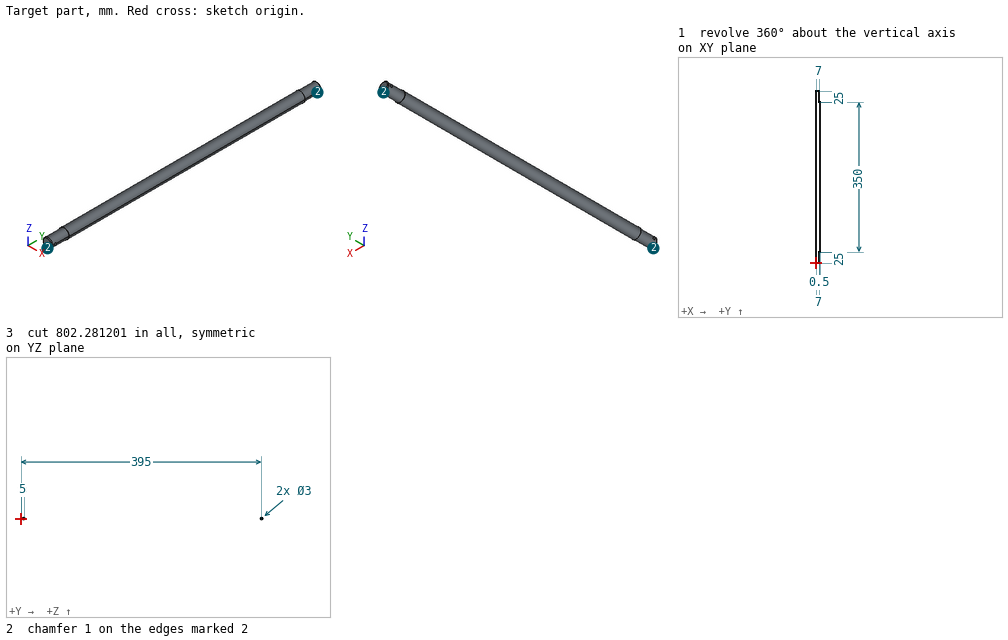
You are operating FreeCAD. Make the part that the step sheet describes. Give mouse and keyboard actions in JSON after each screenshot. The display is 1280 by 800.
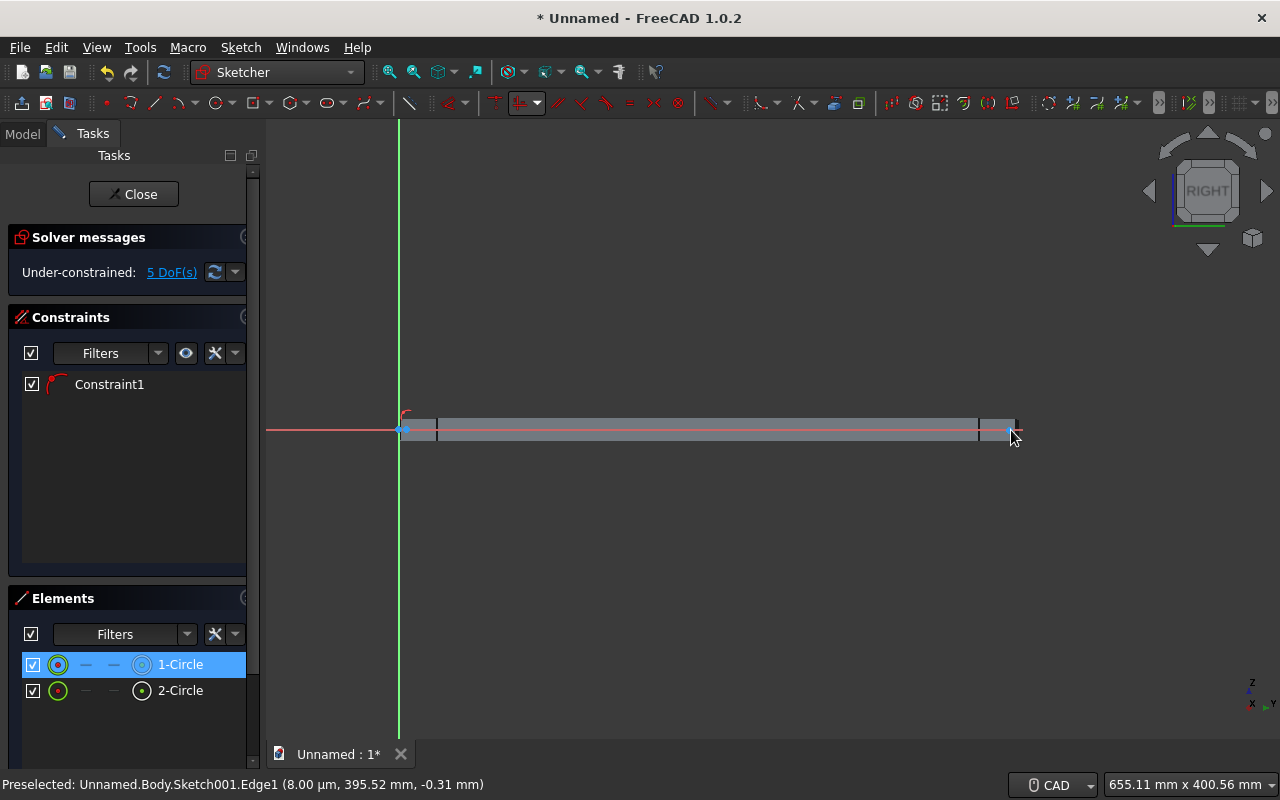
{"action": "scroll", "coordinate": [408, 428], "scroll_direction": "up", "scroll_amount": 12}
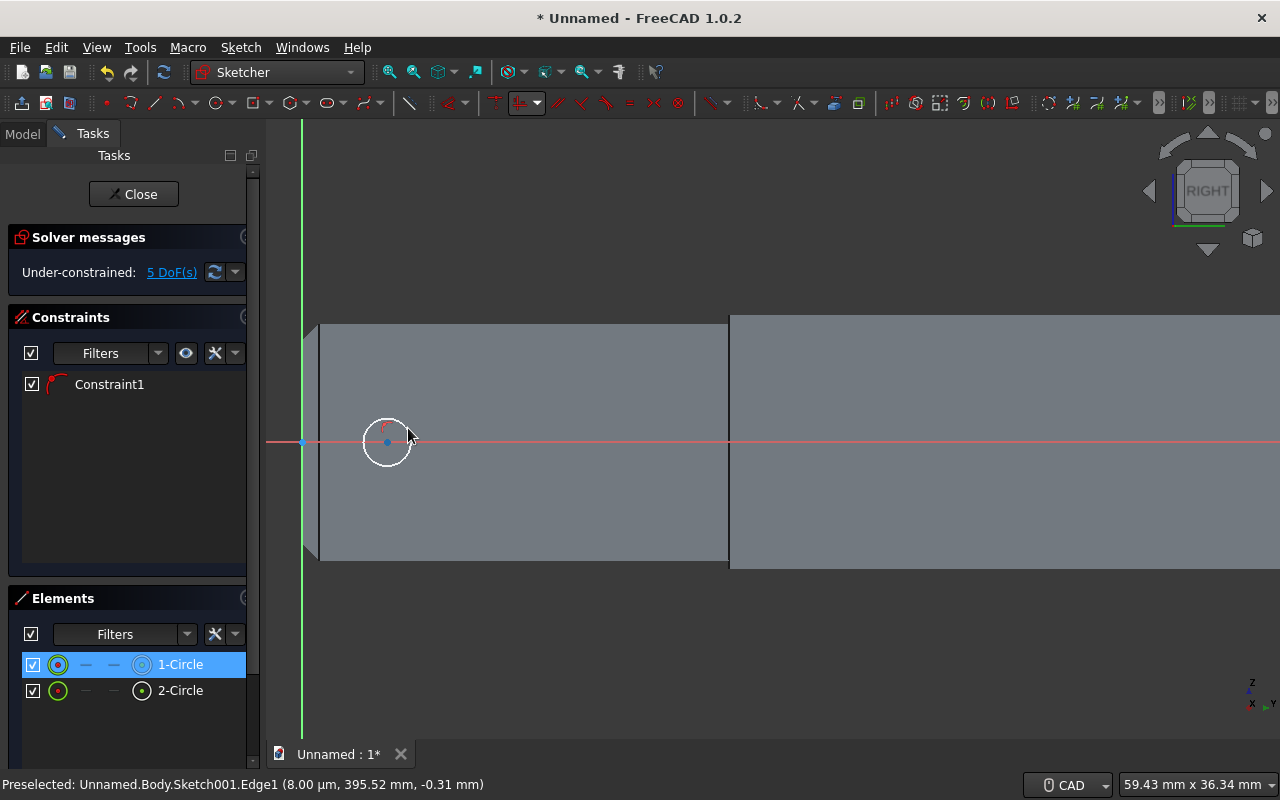
{"action": "left_click", "coordinate": [404, 425]}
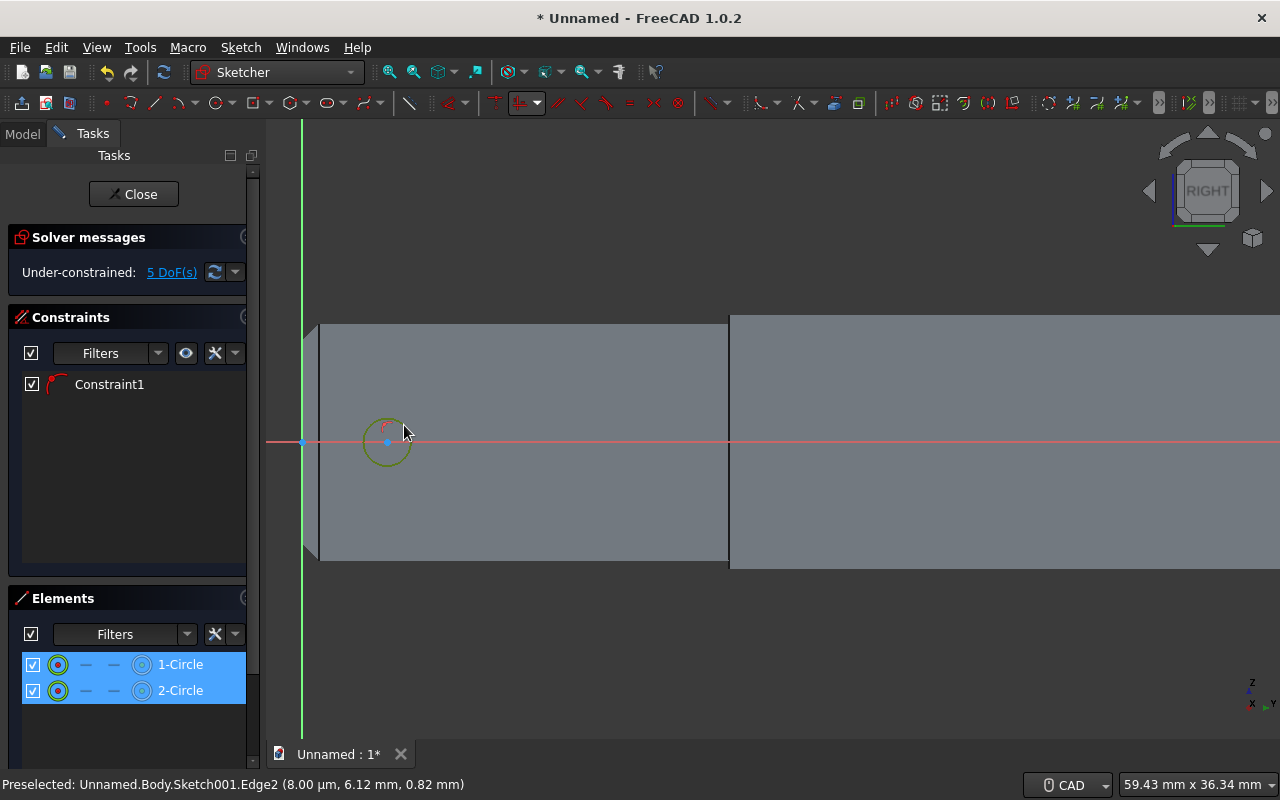
{"action": "left_click", "coordinate": [630, 104]}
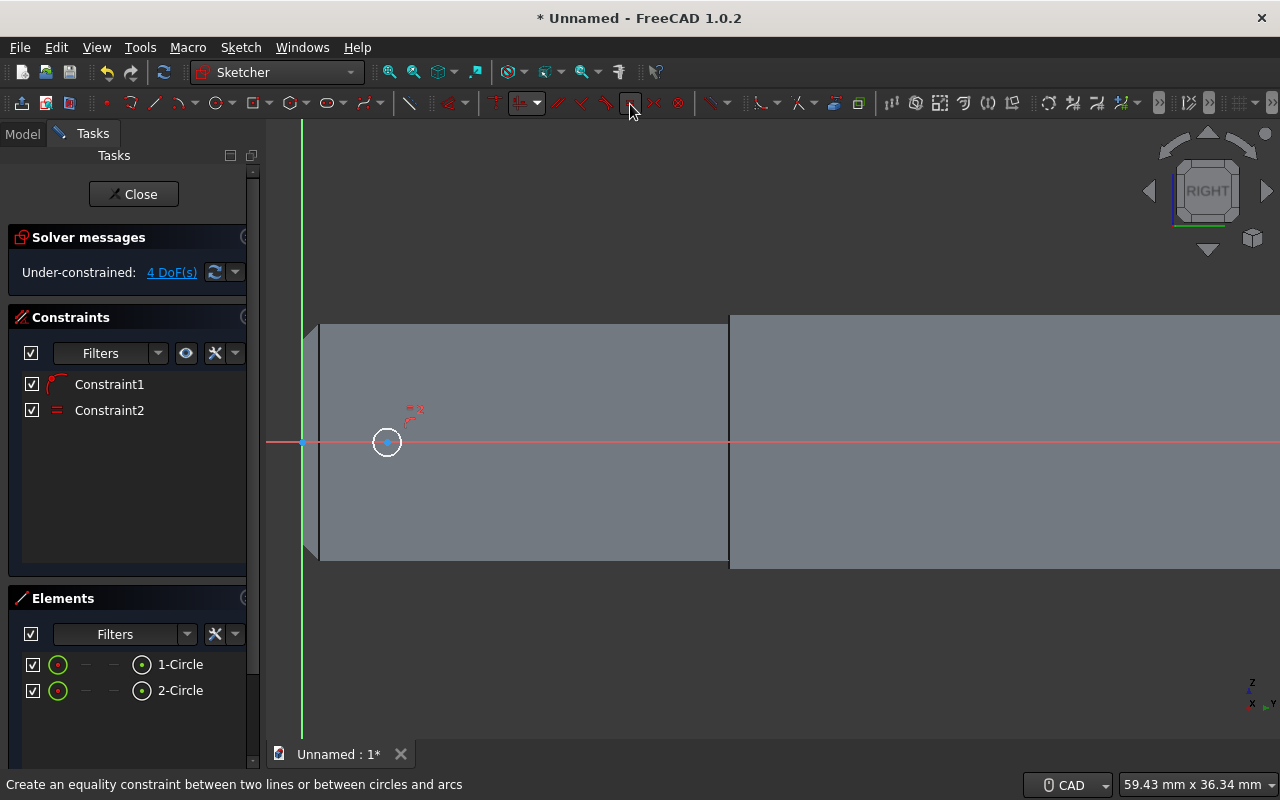
{"action": "scroll", "coordinate": [407, 428], "scroll_direction": "down", "scroll_amount": 12}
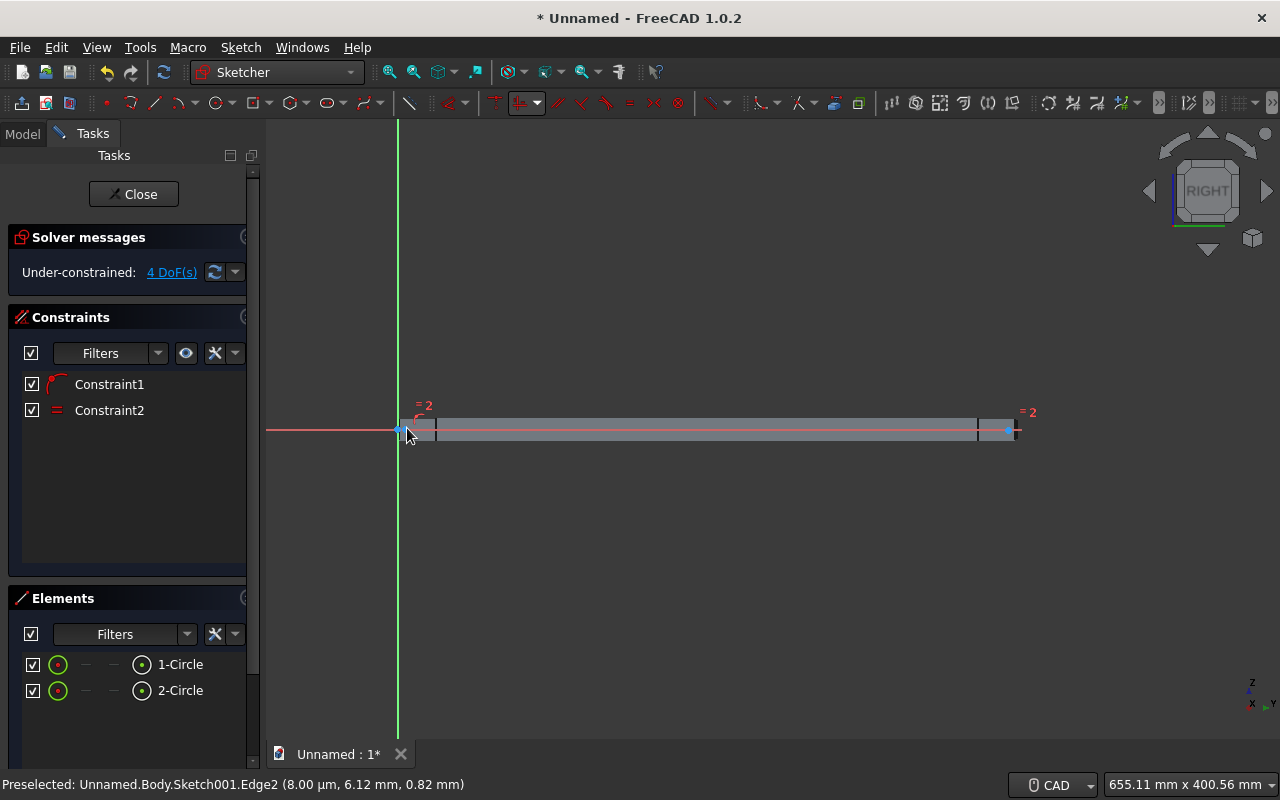
{"action": "left_click", "coordinate": [1009, 431]}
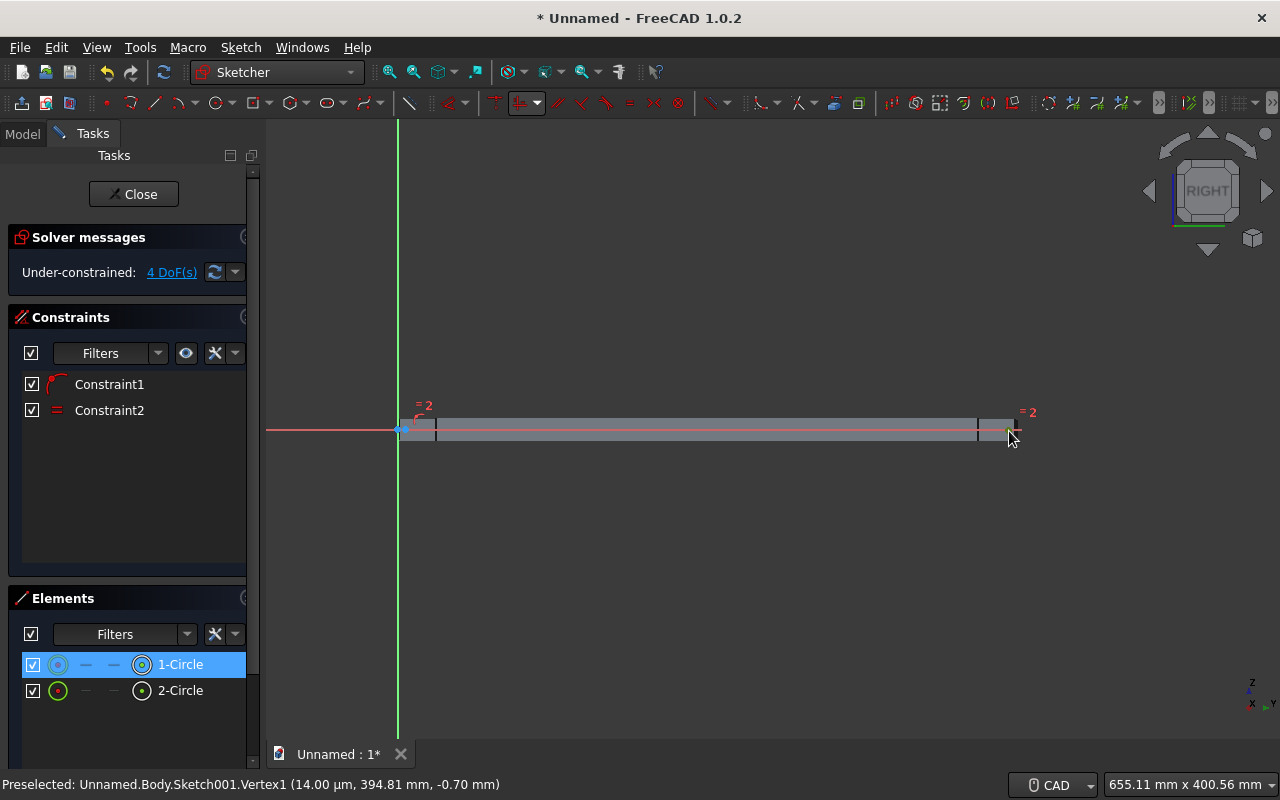
{"action": "left_click", "coordinate": [353, 430]}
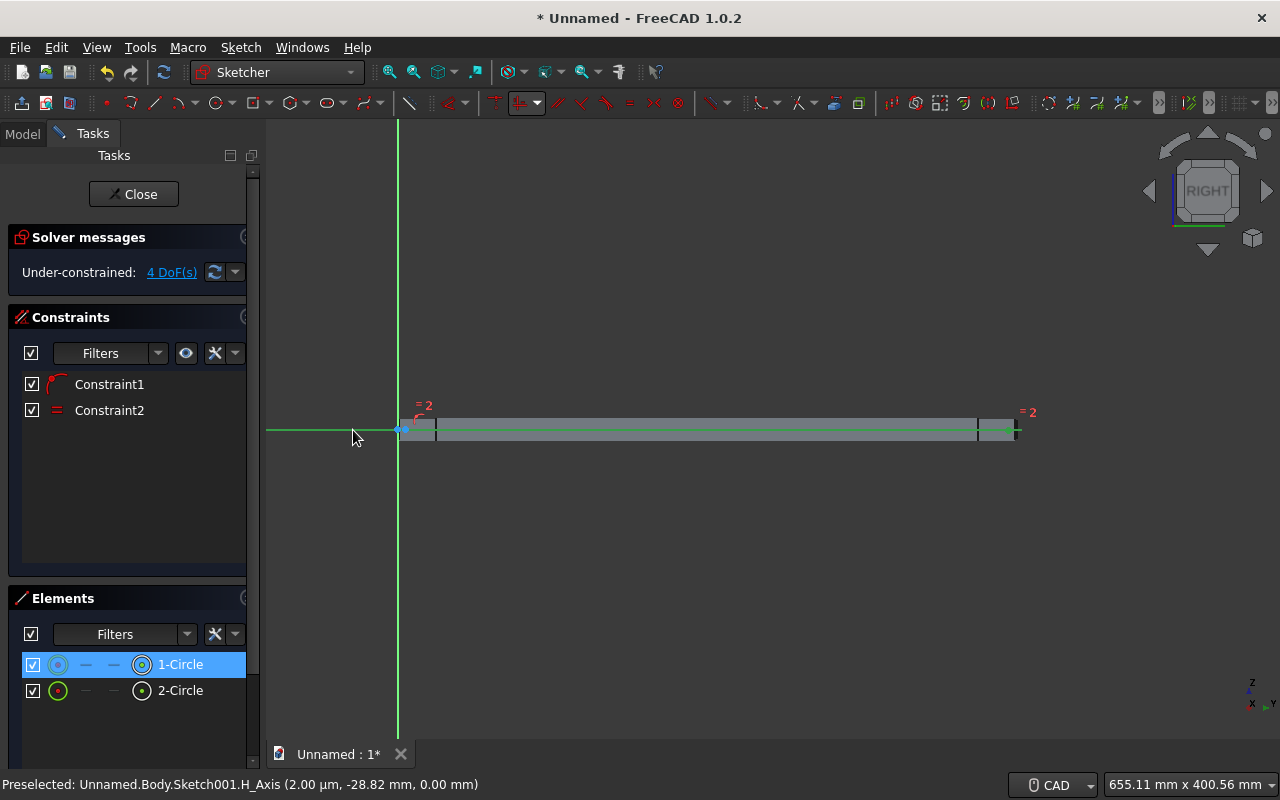
{"action": "key", "text": "c"}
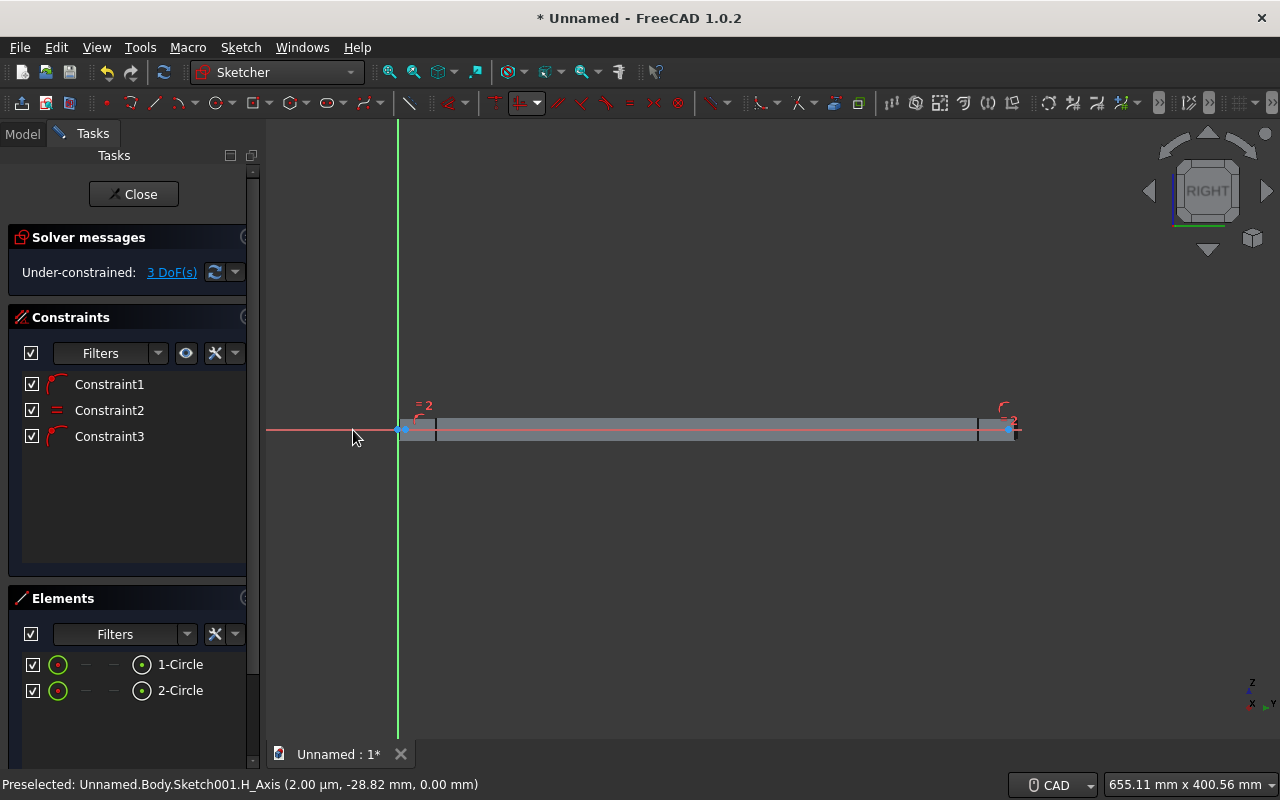
{"action": "left_click", "coordinate": [448, 104]}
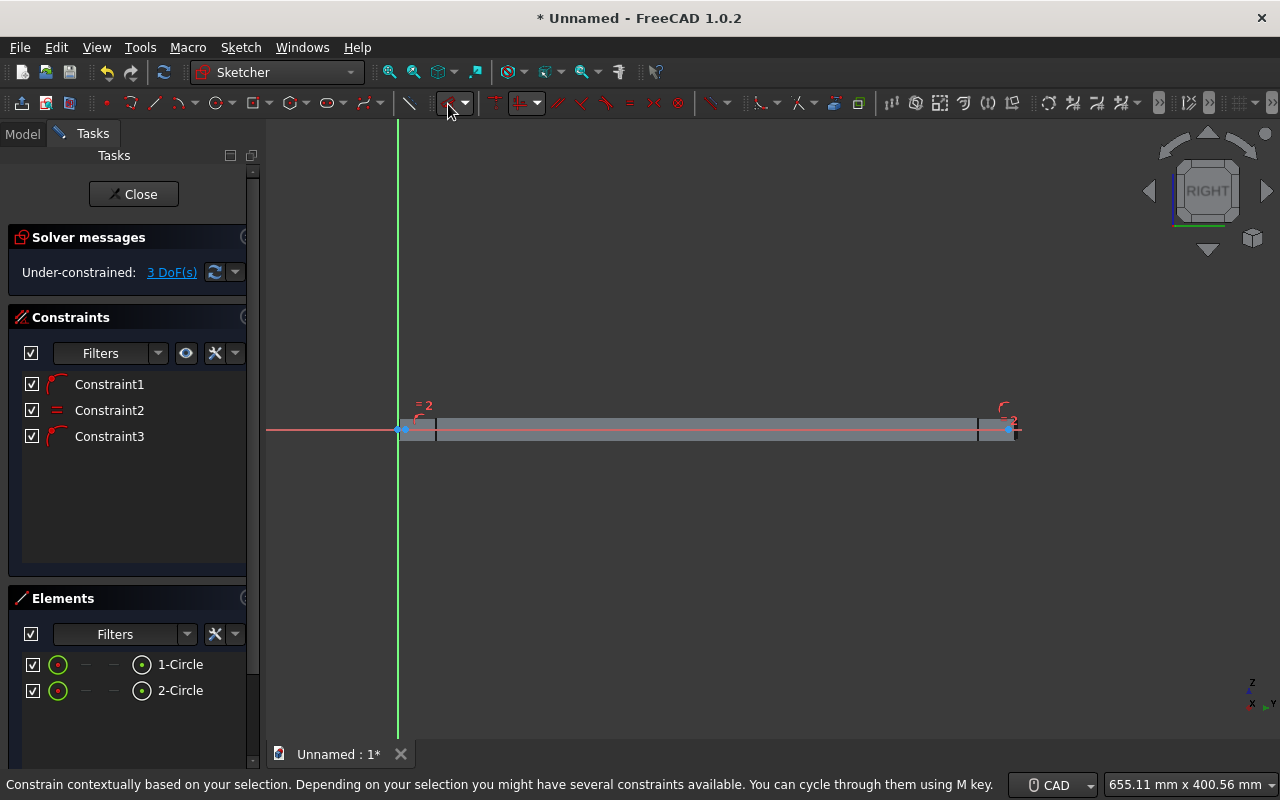
{"action": "scroll", "coordinate": [1007, 430], "scroll_direction": "up", "scroll_amount": 13}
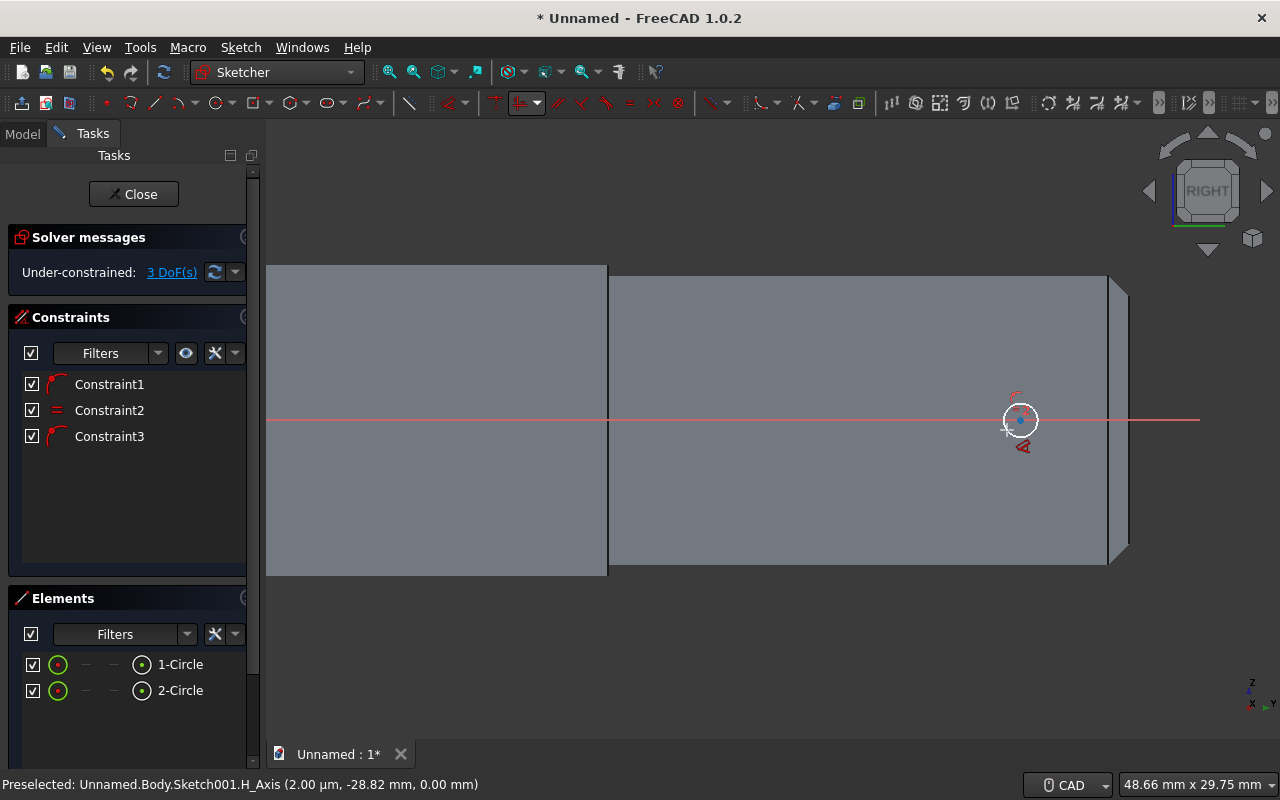
{"action": "left_click", "coordinate": [1004, 420]}
{"action": "left_click", "coordinate": [979, 396]}